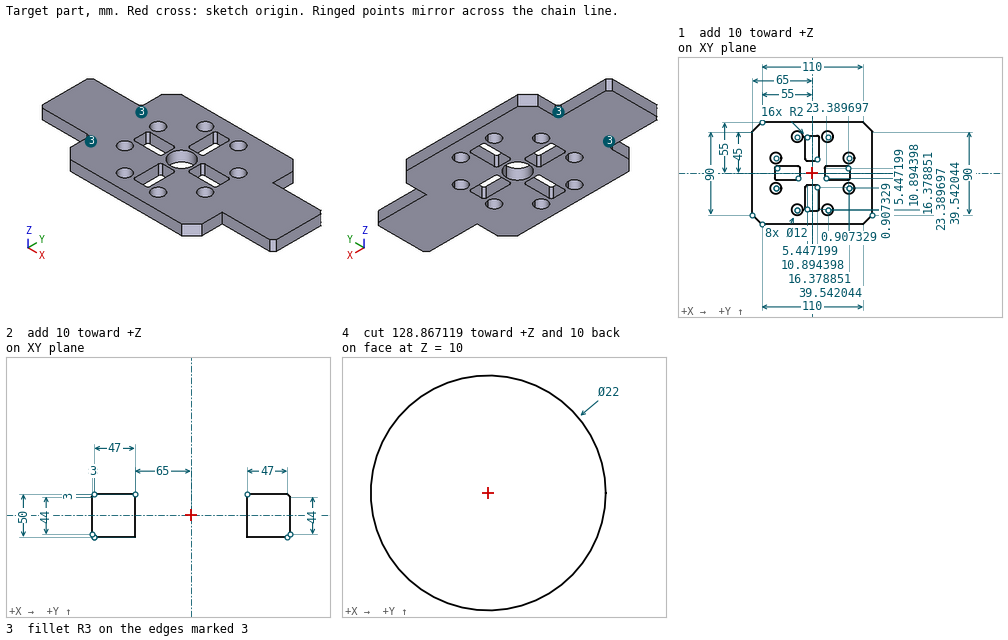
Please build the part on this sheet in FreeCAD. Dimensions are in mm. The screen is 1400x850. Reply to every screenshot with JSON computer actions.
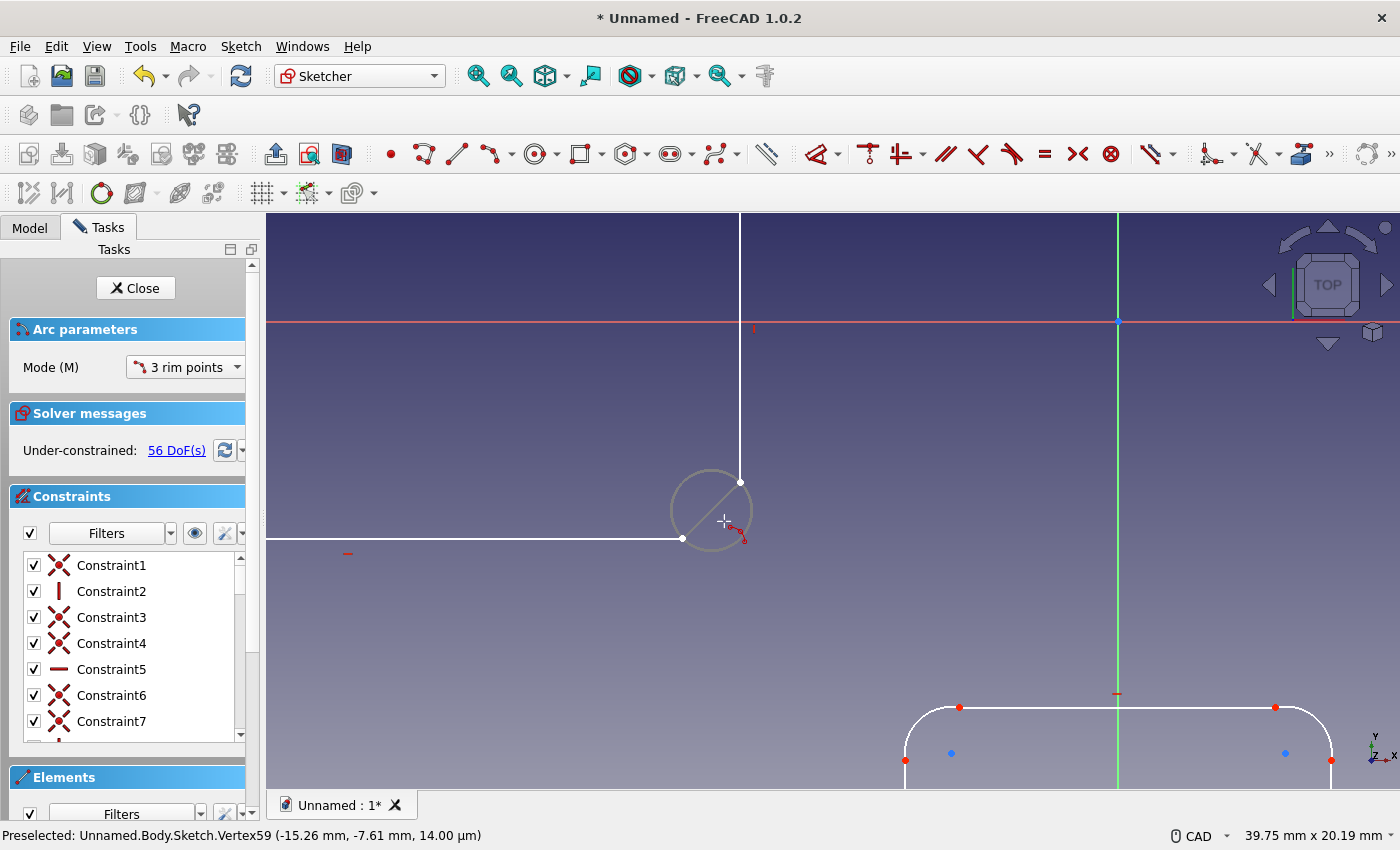
{"action": "left_click", "coordinate": [724, 517]}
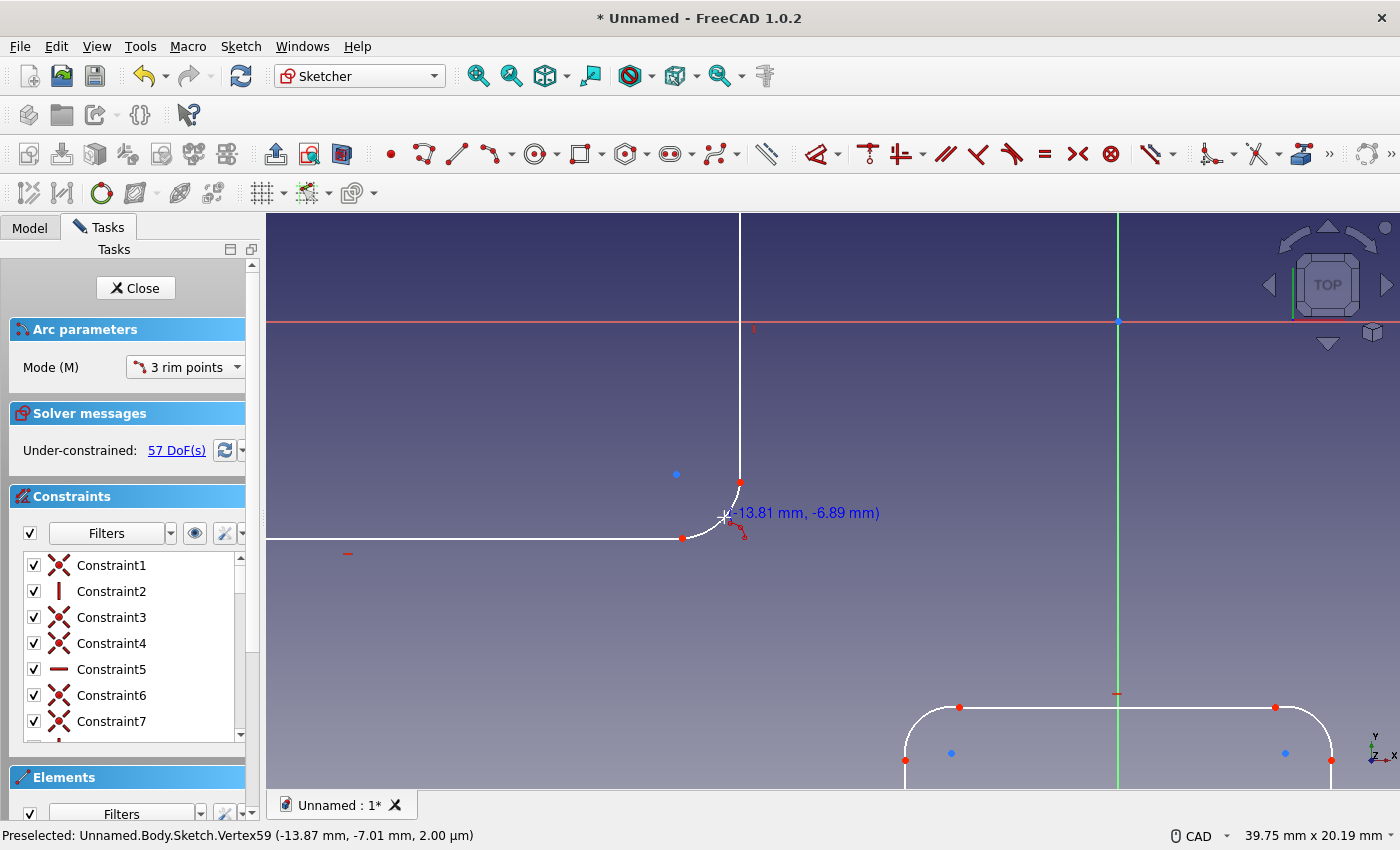
{"action": "scroll", "coordinate": [720, 523], "scroll_direction": "down", "scroll_amount": 11}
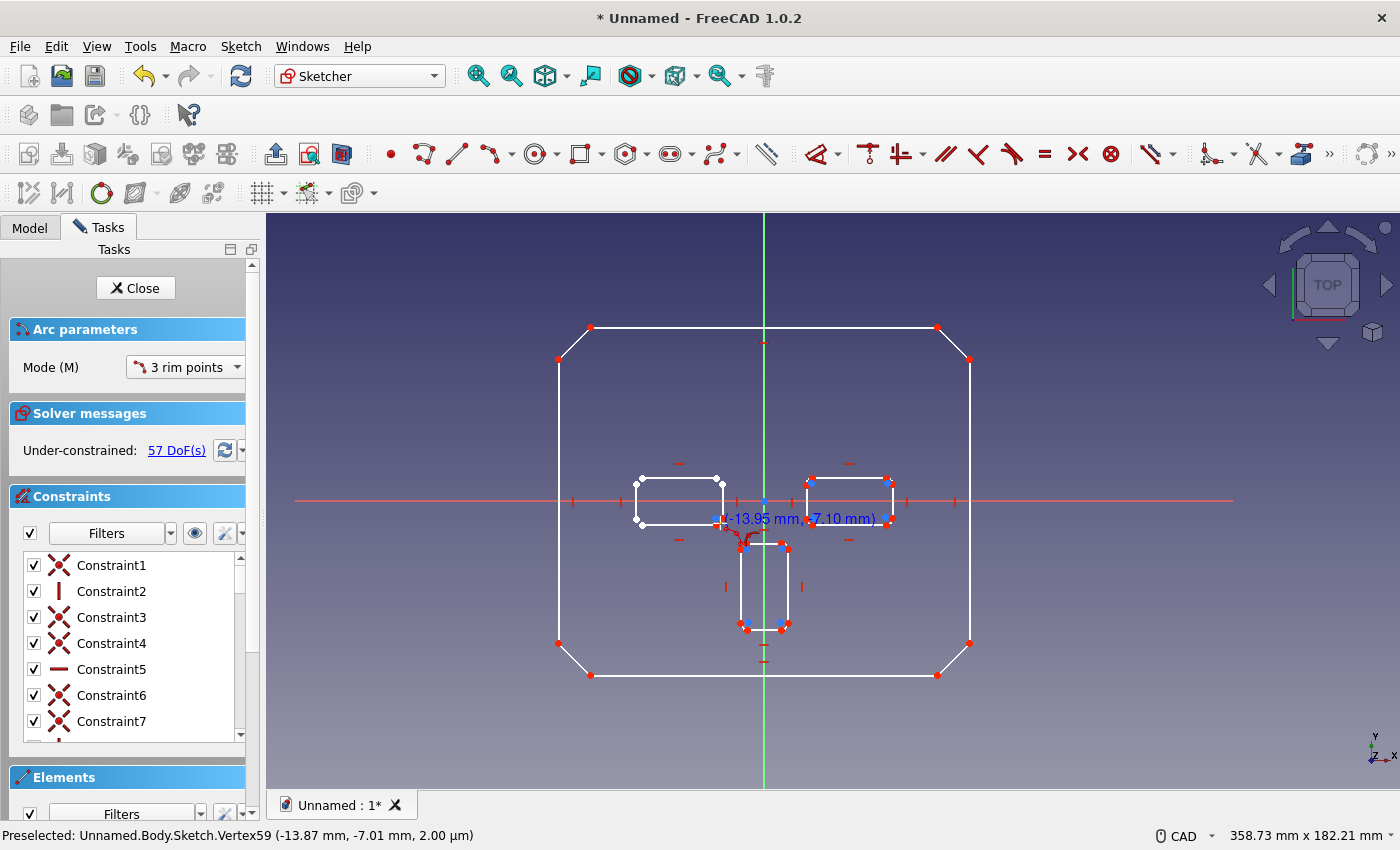
{"action": "scroll", "coordinate": [642, 525], "scroll_direction": "up", "scroll_amount": 3}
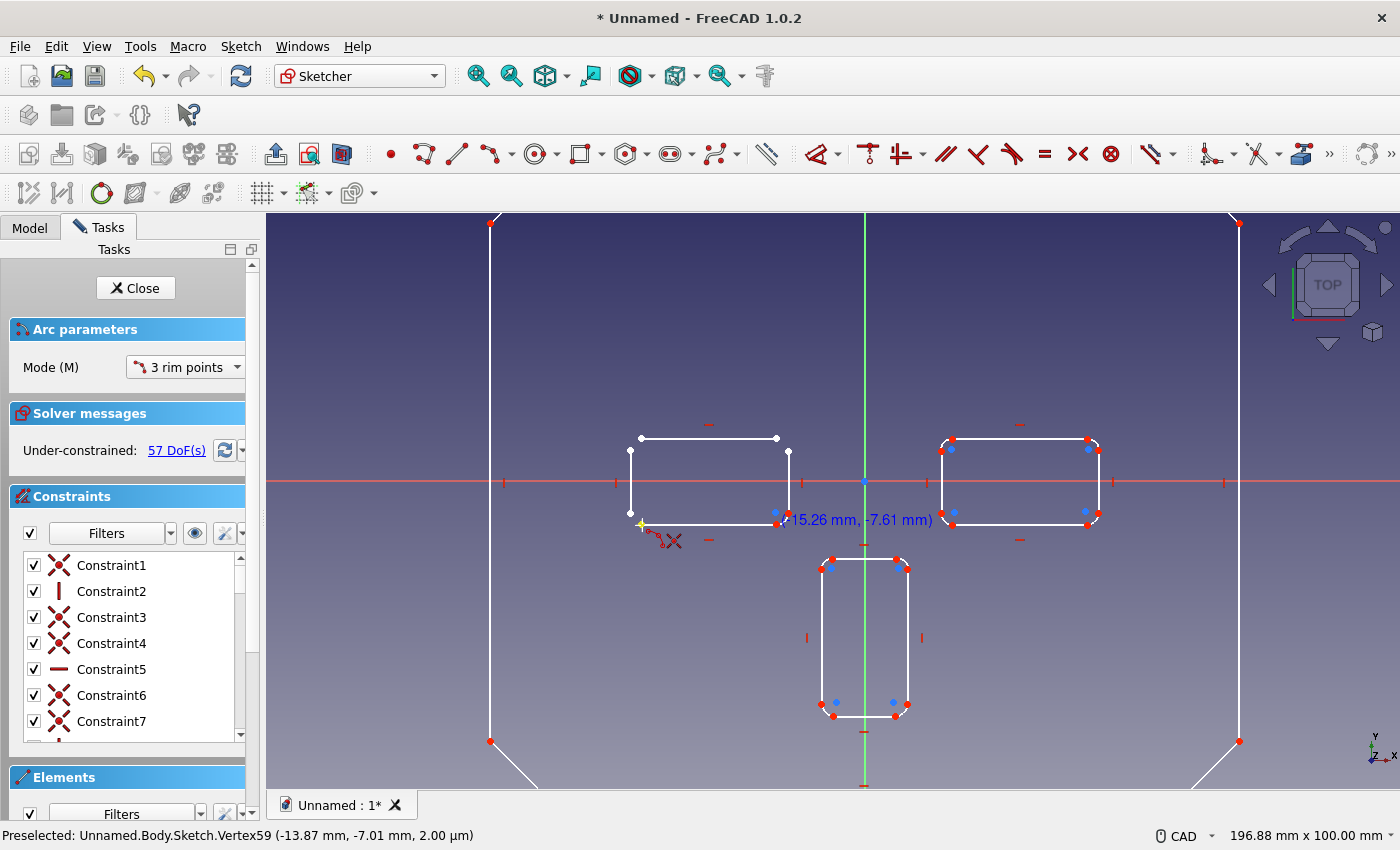
{"action": "left_click", "coordinate": [642, 525]}
{"action": "left_click", "coordinate": [631, 514]}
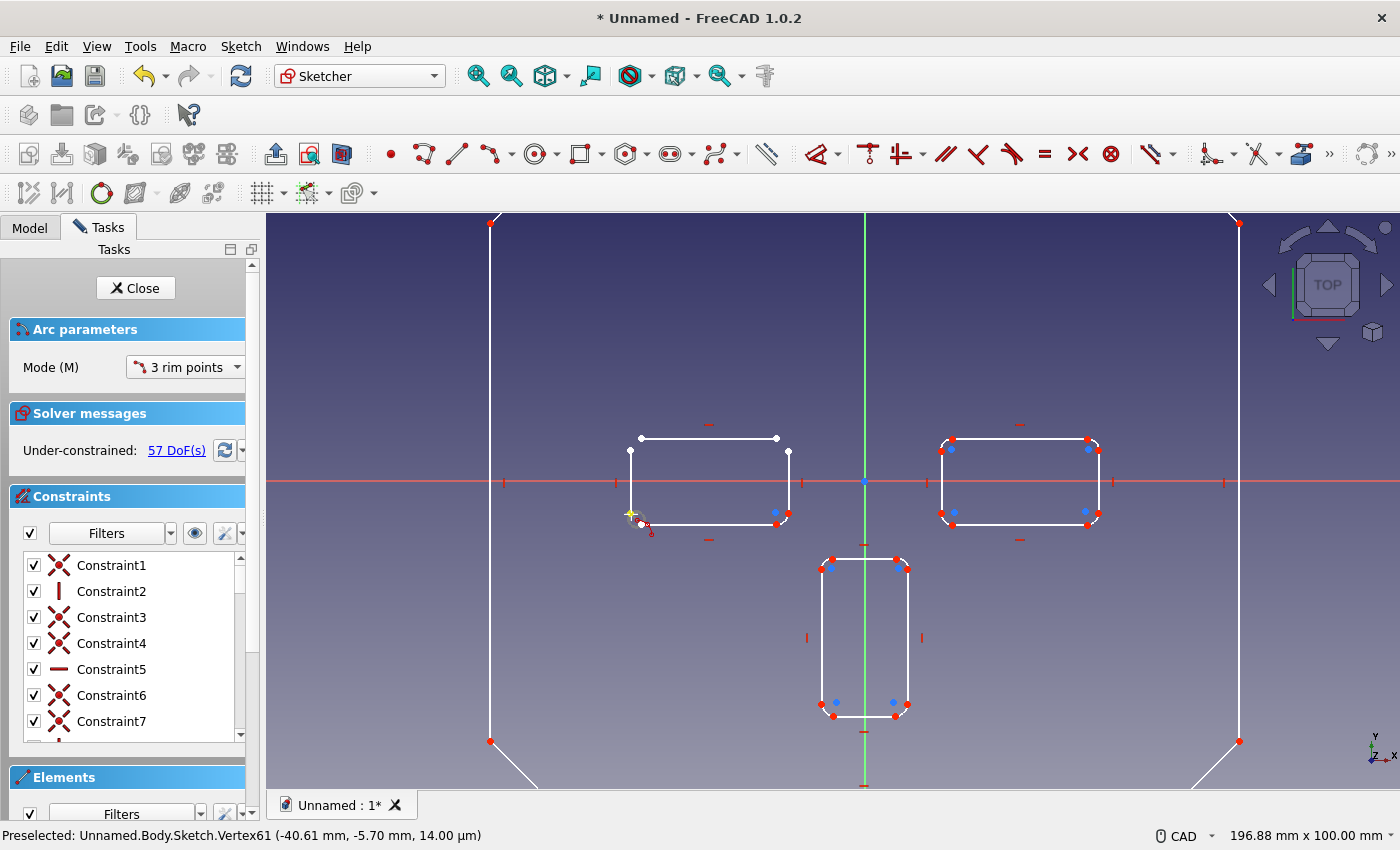
{"action": "scroll", "coordinate": [634, 521], "scroll_direction": "up", "scroll_amount": 8}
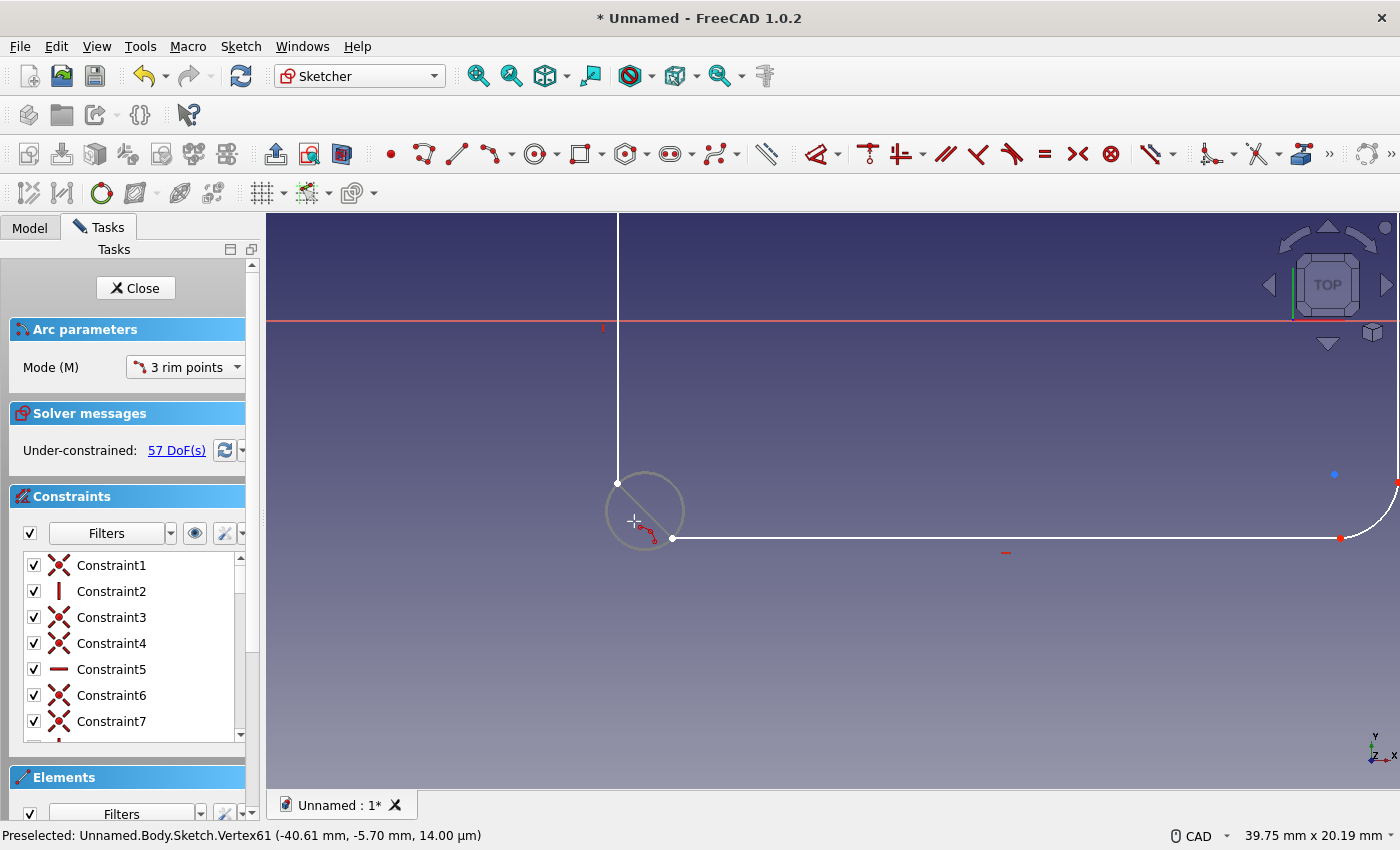
{"action": "left_click", "coordinate": [634, 517]}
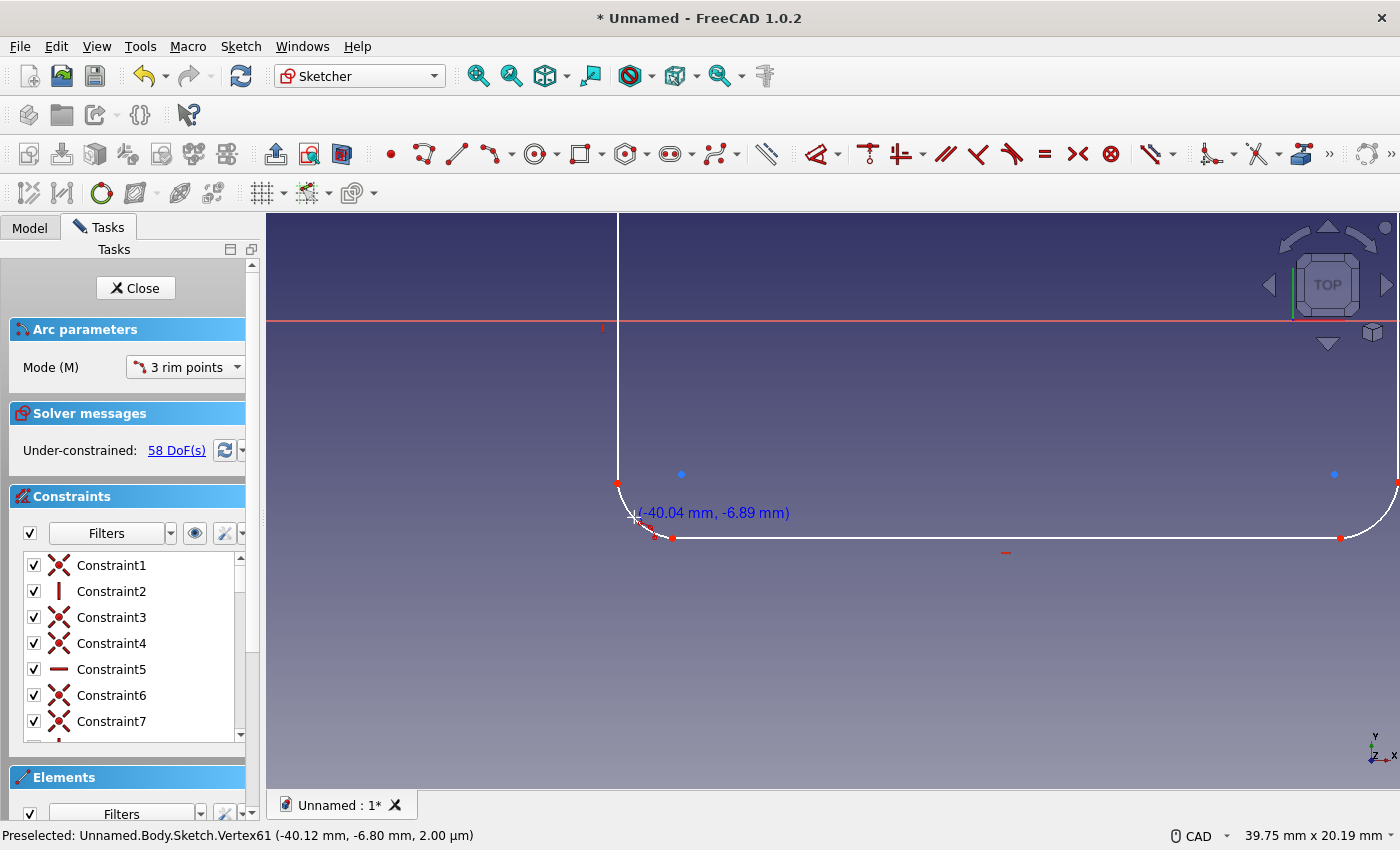
{"action": "scroll", "coordinate": [638, 523], "scroll_direction": "down", "scroll_amount": 11}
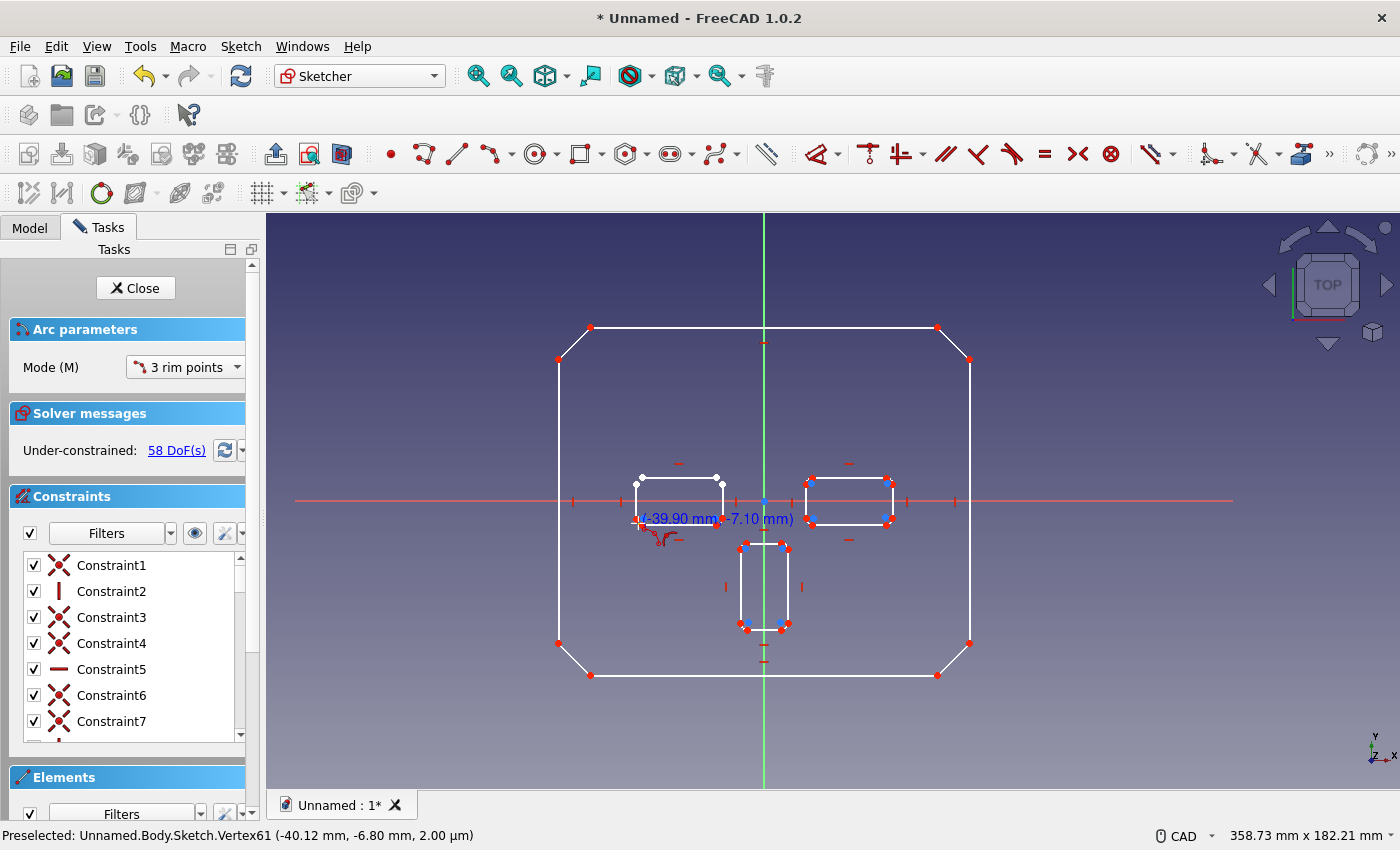
{"action": "scroll", "coordinate": [636, 484], "scroll_direction": "up", "scroll_amount": 3}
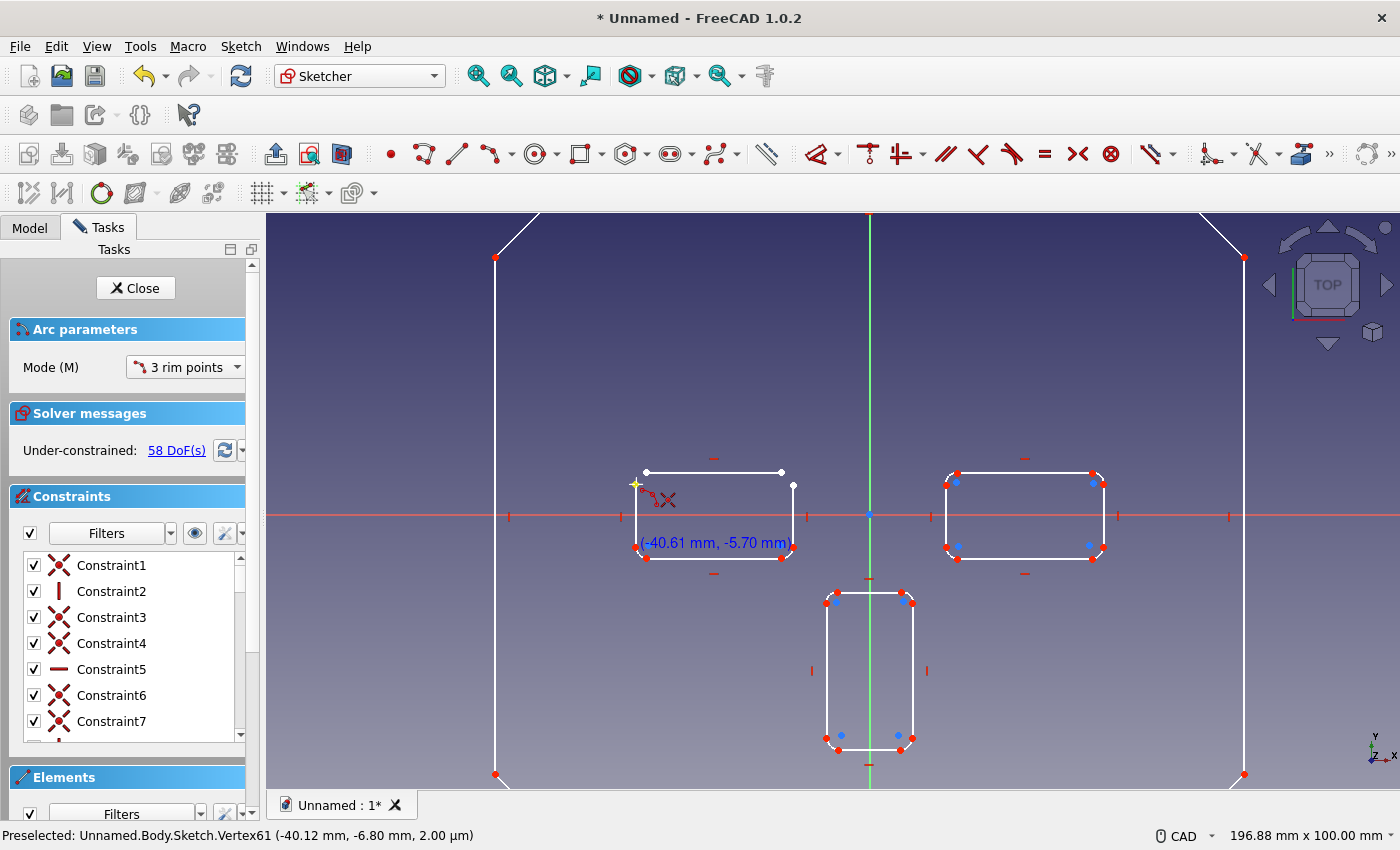
{"action": "left_click", "coordinate": [636, 485]}
{"action": "left_click", "coordinate": [647, 473]}